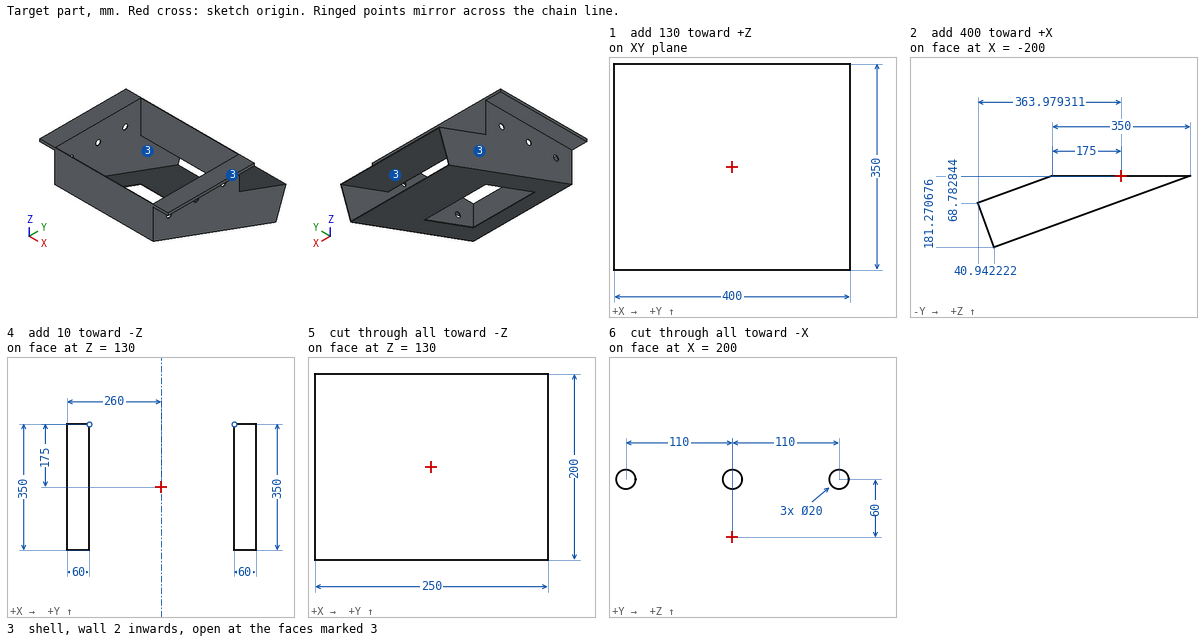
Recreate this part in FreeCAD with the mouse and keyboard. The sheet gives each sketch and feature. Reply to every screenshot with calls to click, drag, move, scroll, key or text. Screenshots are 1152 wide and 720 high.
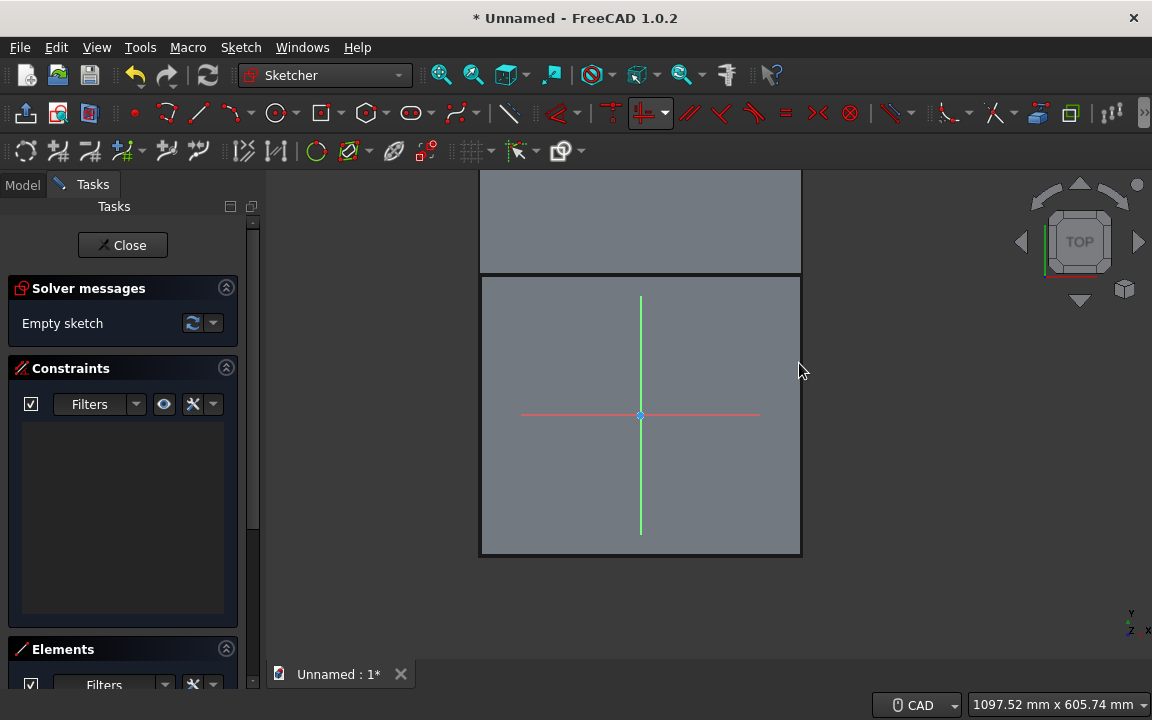
key(g)
key(r)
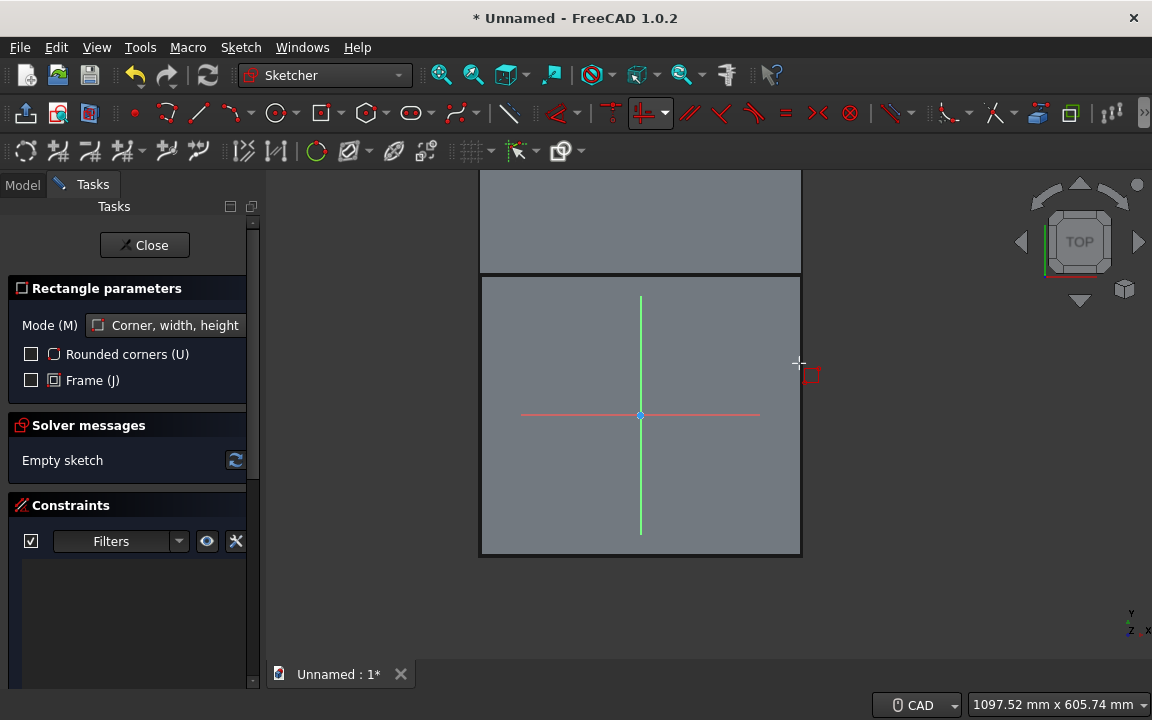
click(431, 274)
move(479, 557)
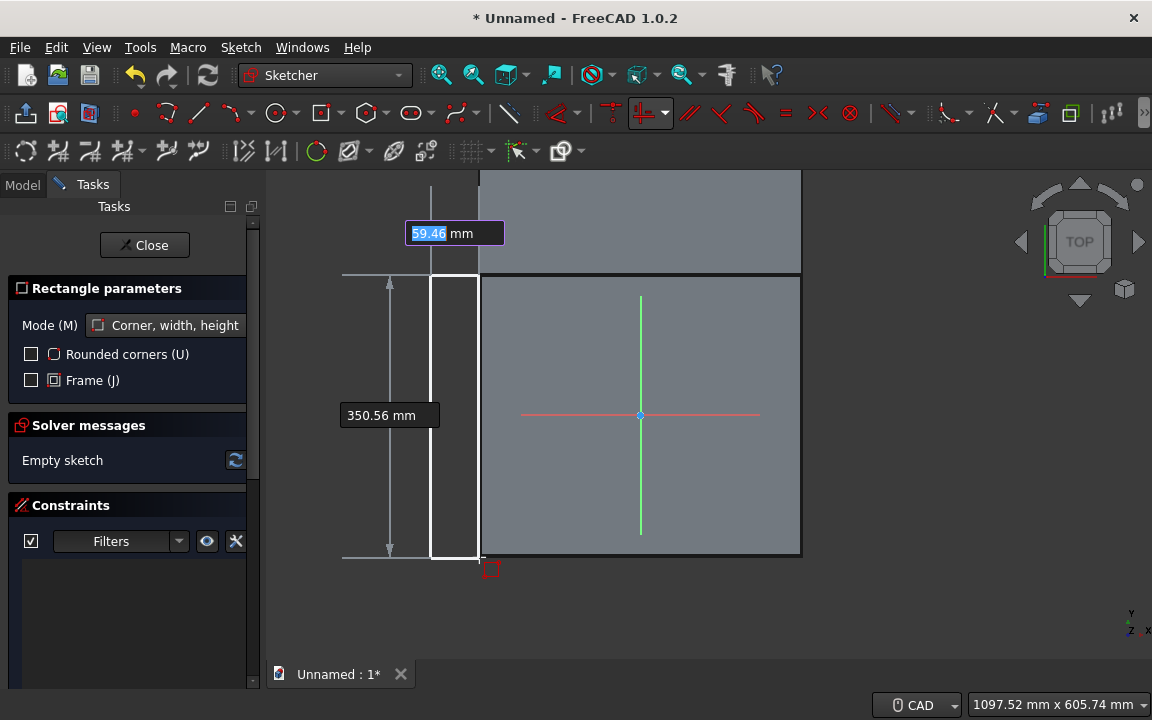
text(60)
key(Tab)
text(350)
key(Return)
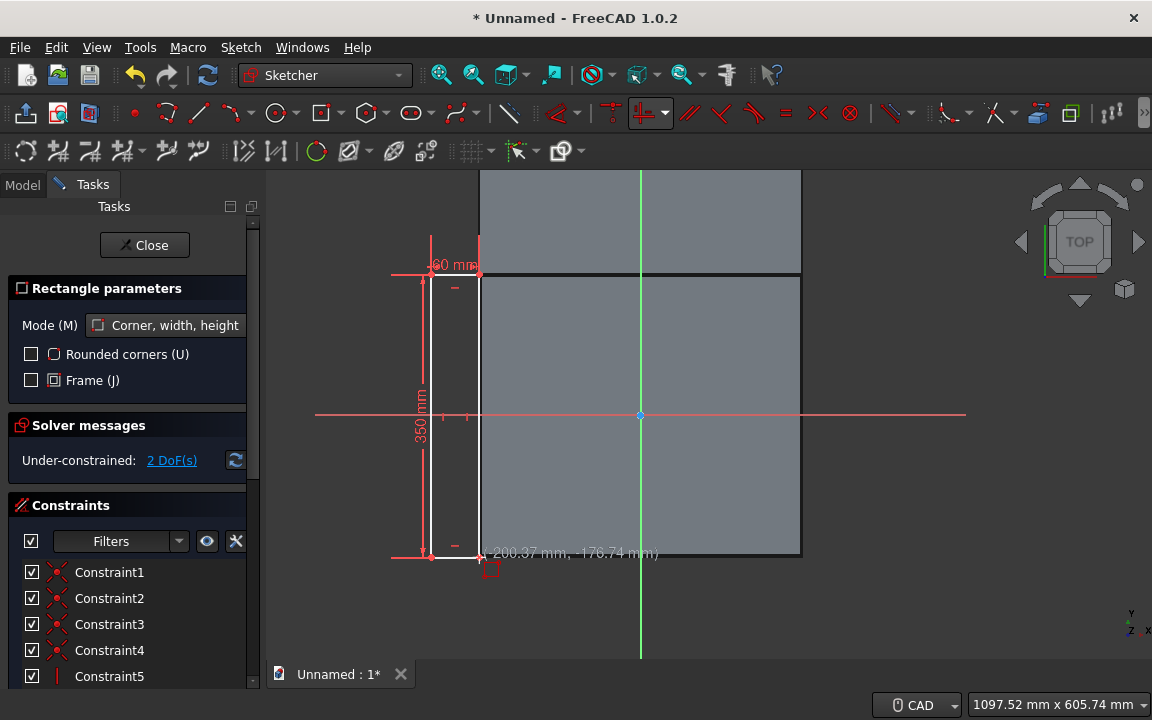
click(802, 274)
move(851, 557)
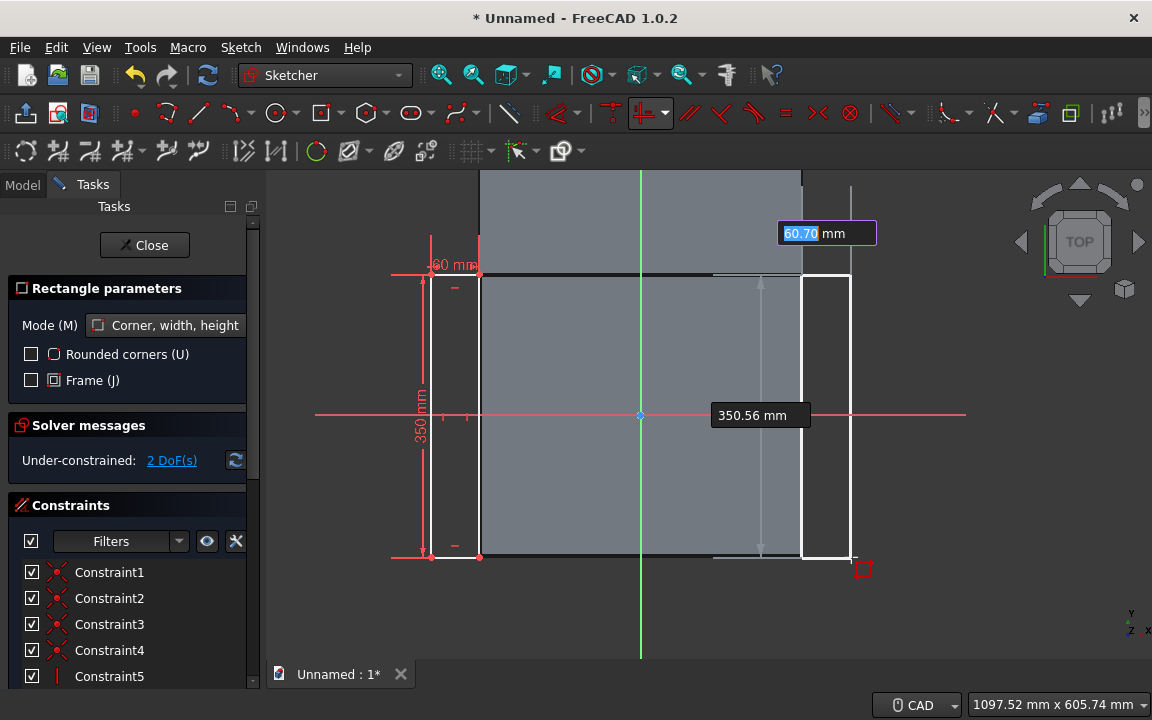
text(60)
key(Tab)
text(350)
key(Return)
key(Escape)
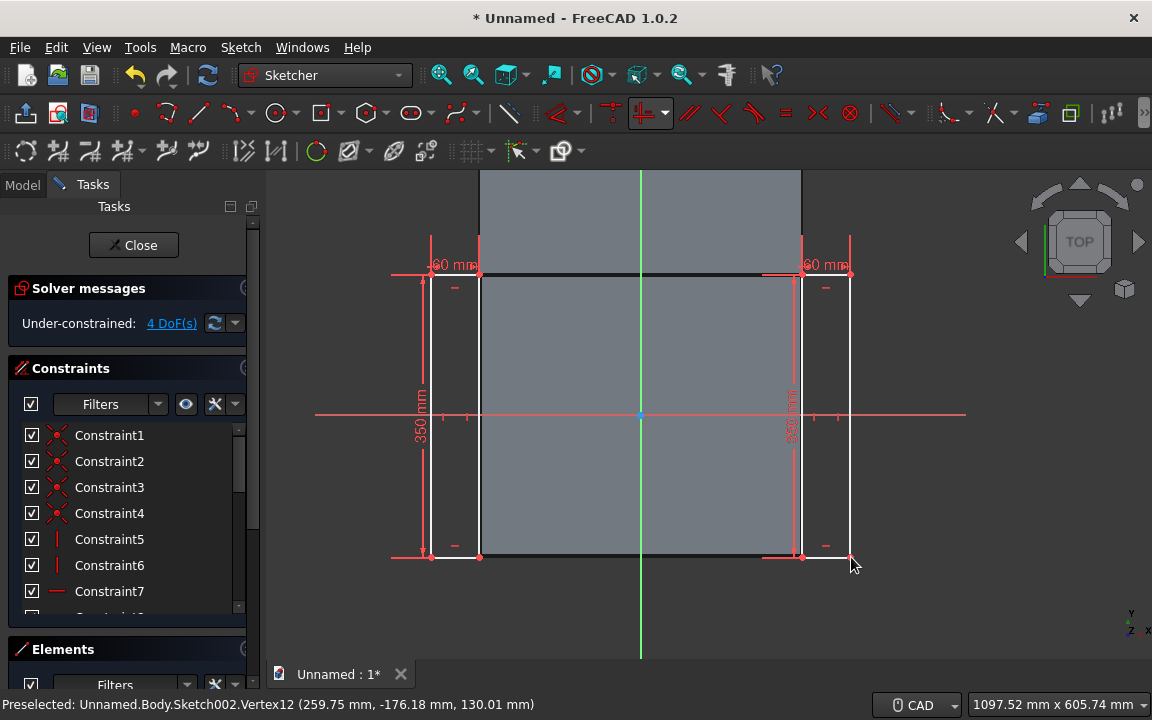
click(479, 275)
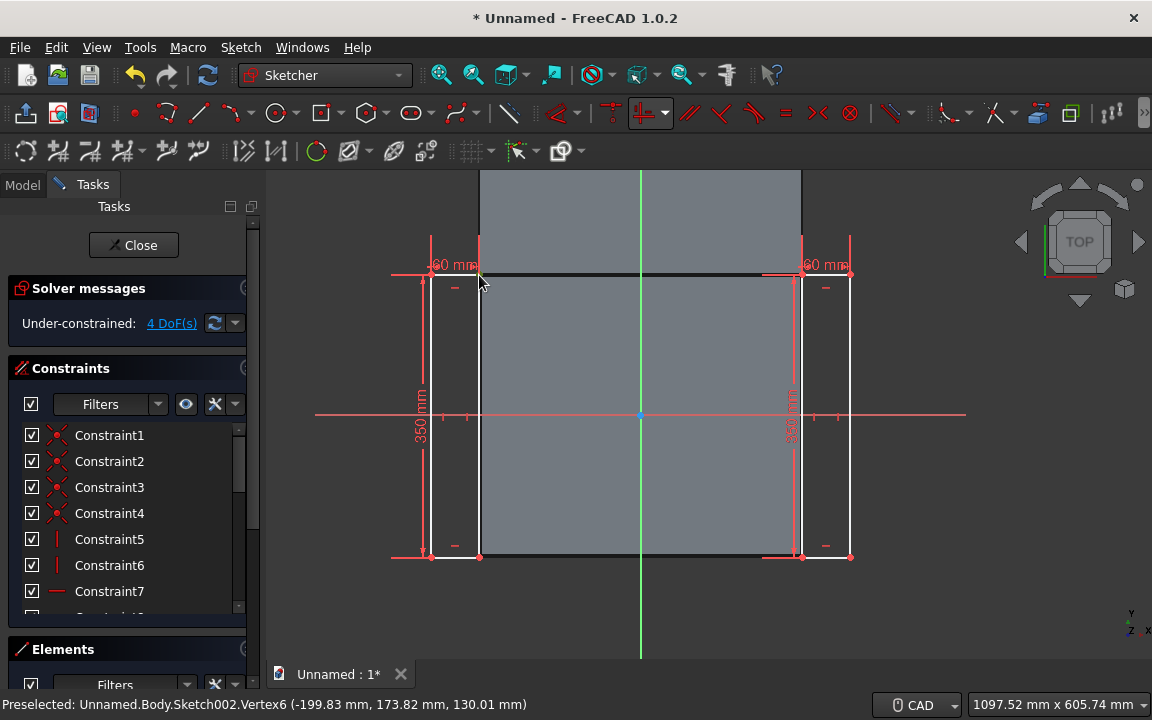
click(802, 275)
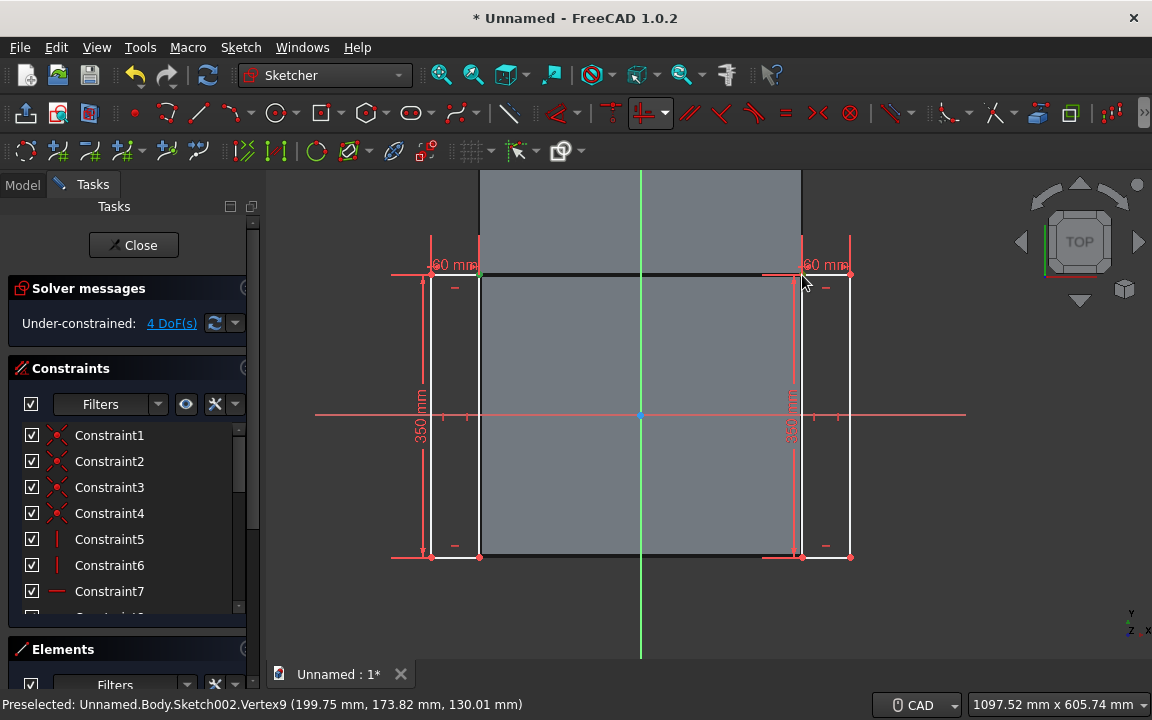
click(641, 600)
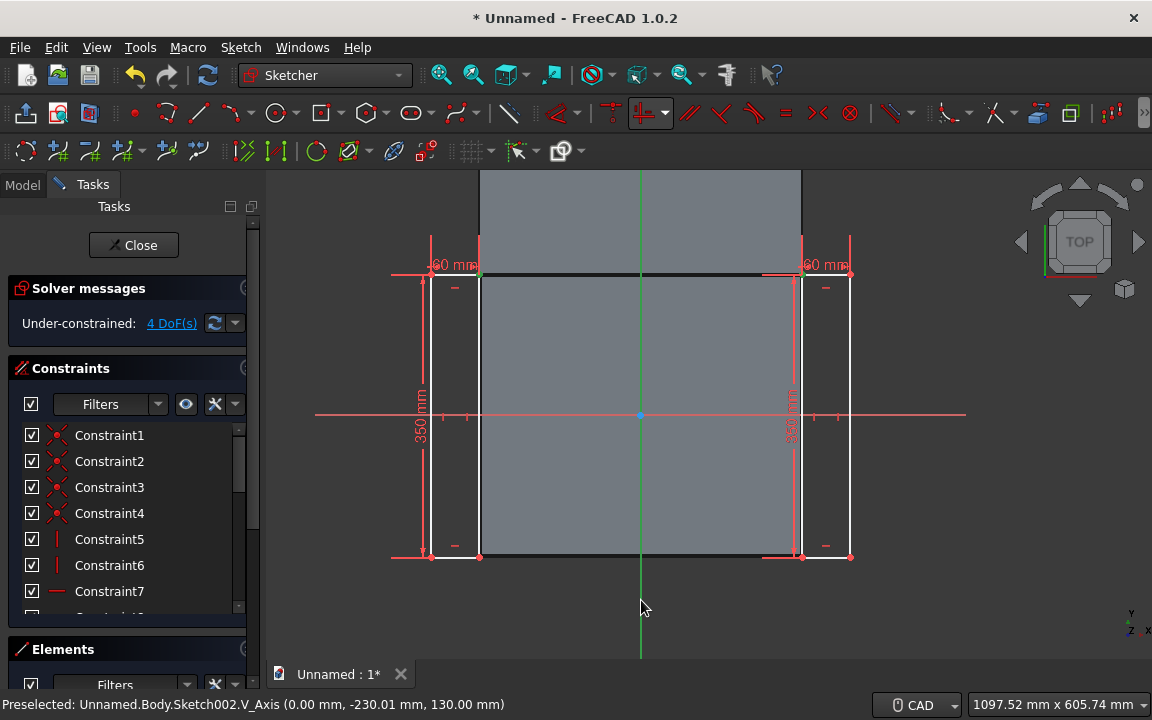
click(818, 114)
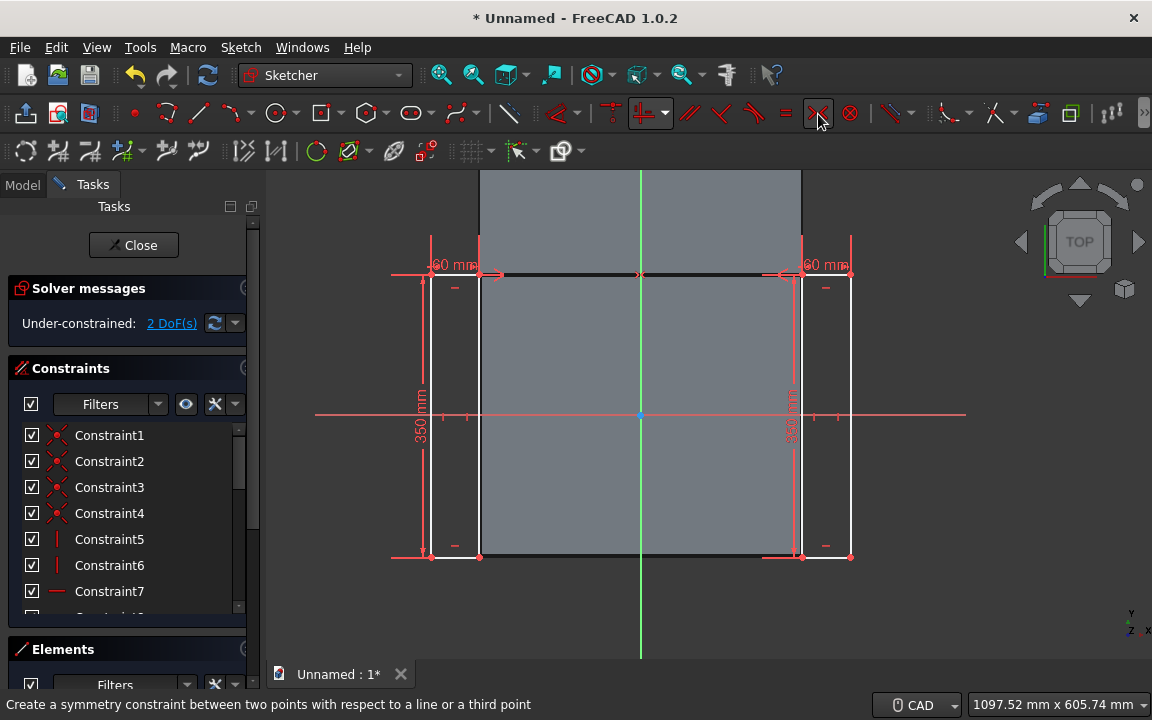
click(431, 275)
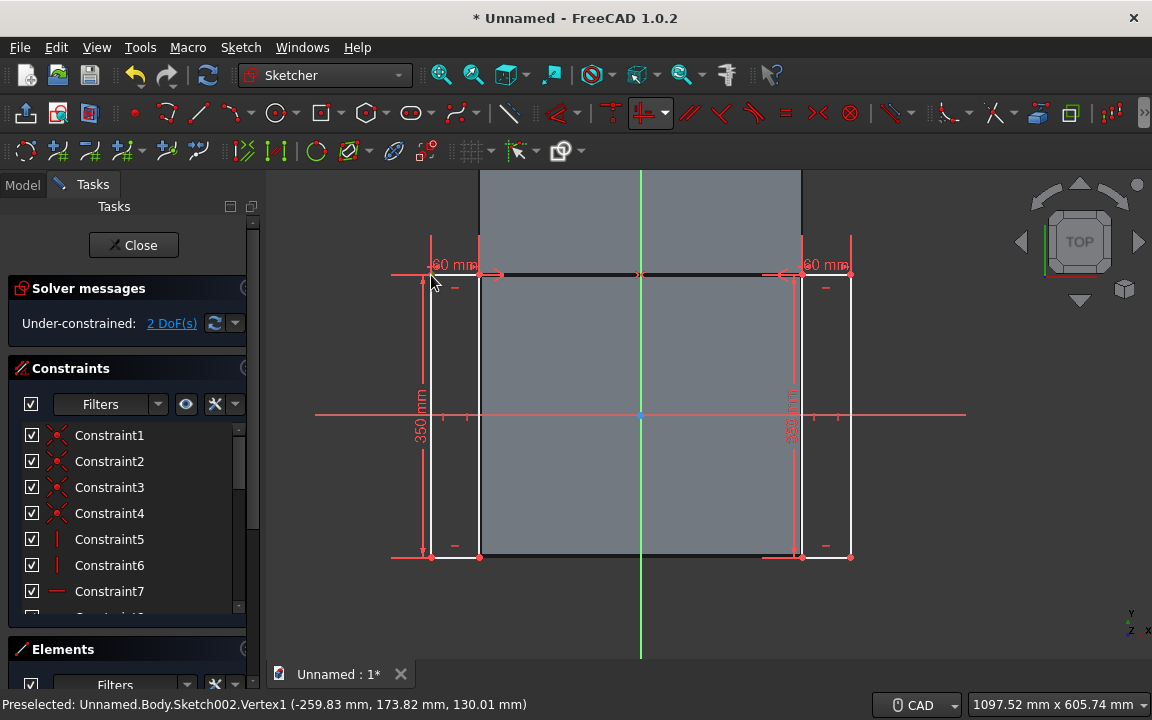
key(l)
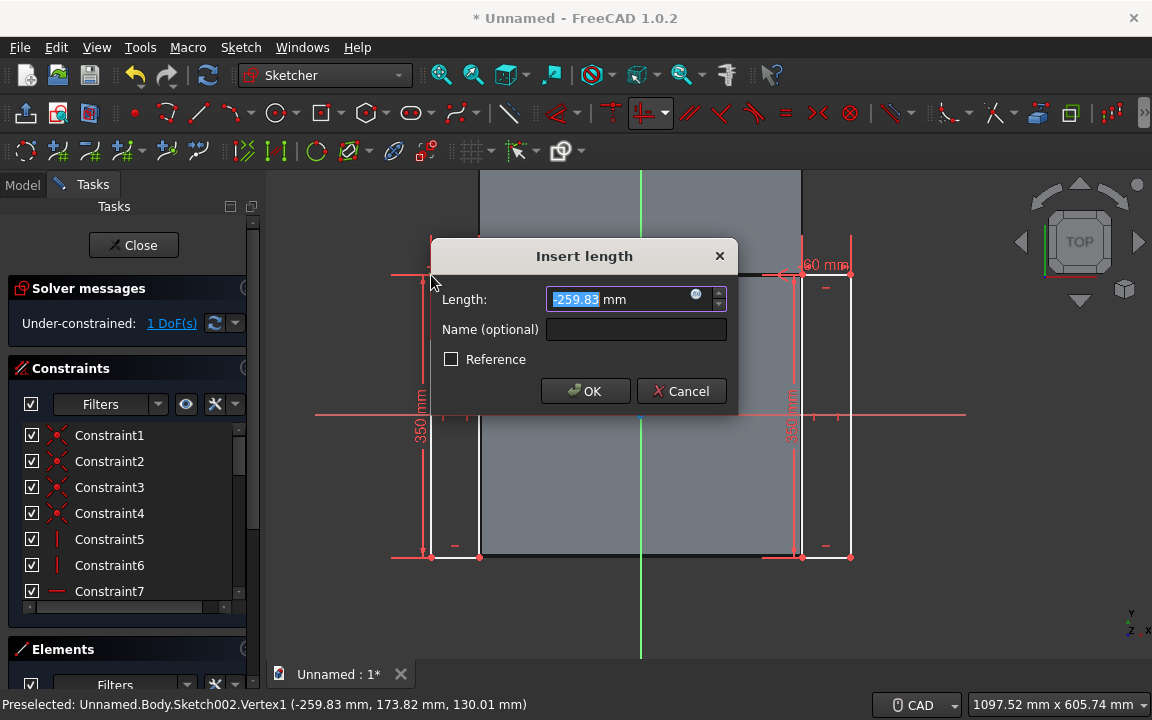
text(-260)
key(Return)